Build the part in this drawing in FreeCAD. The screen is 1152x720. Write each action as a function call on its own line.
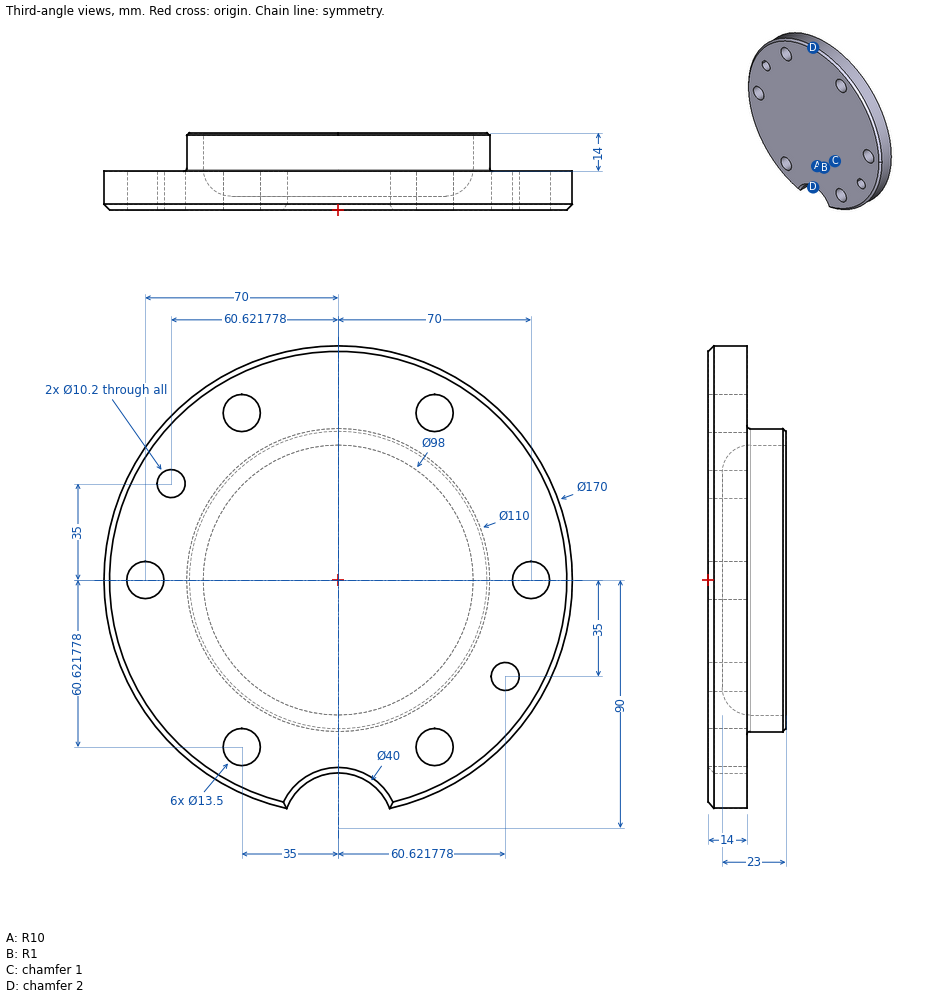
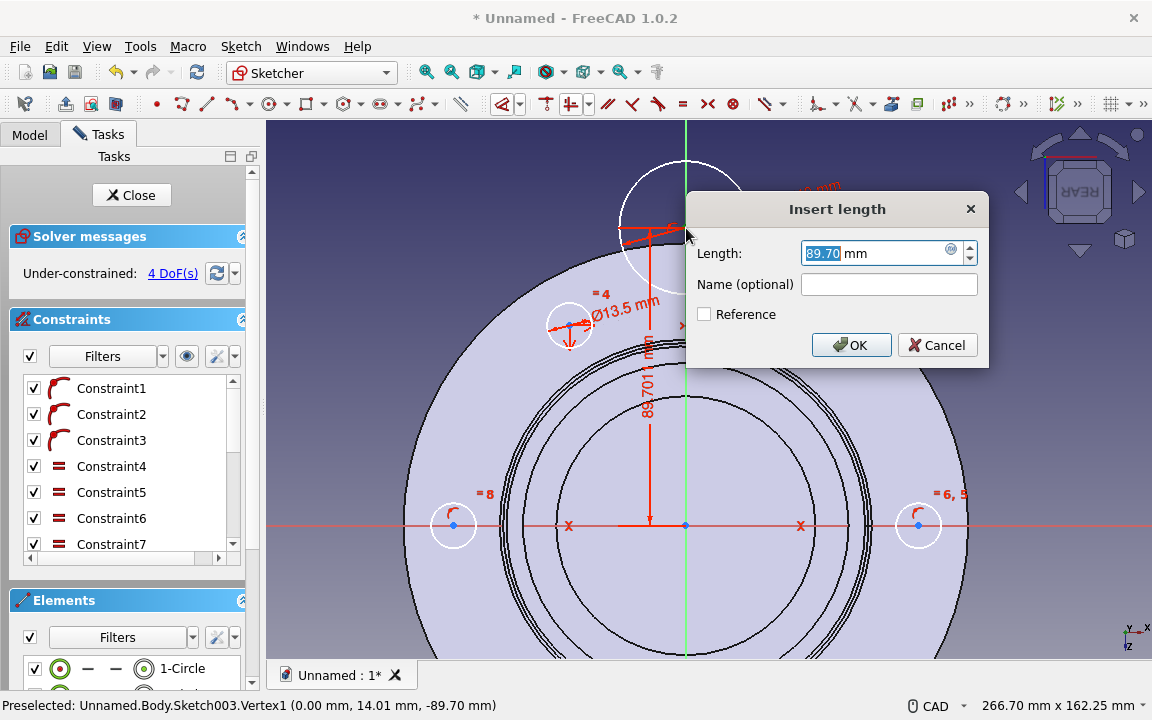
text(90)
key(Return)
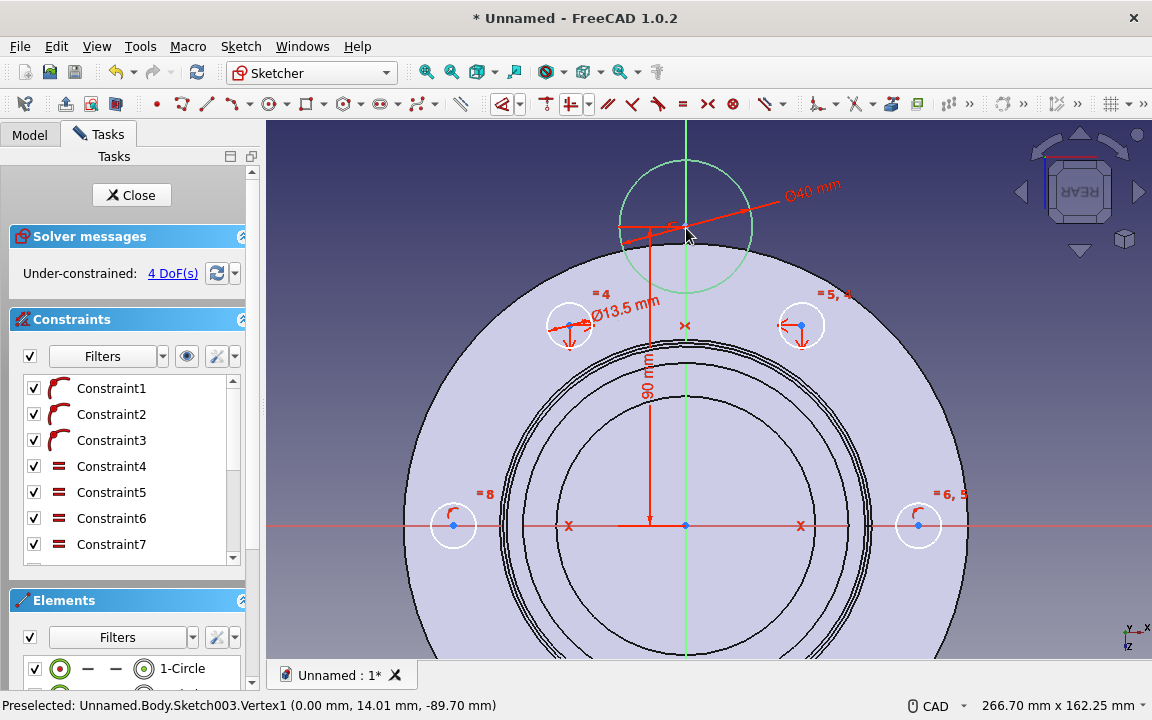
click(570, 325)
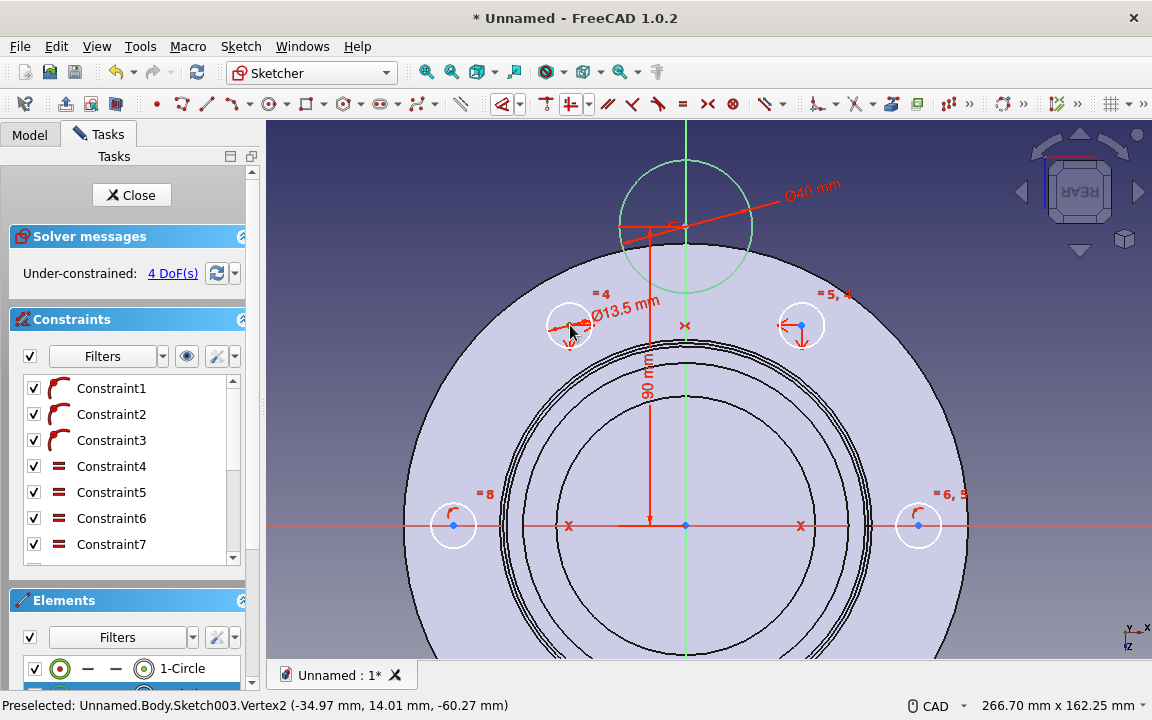
key(l)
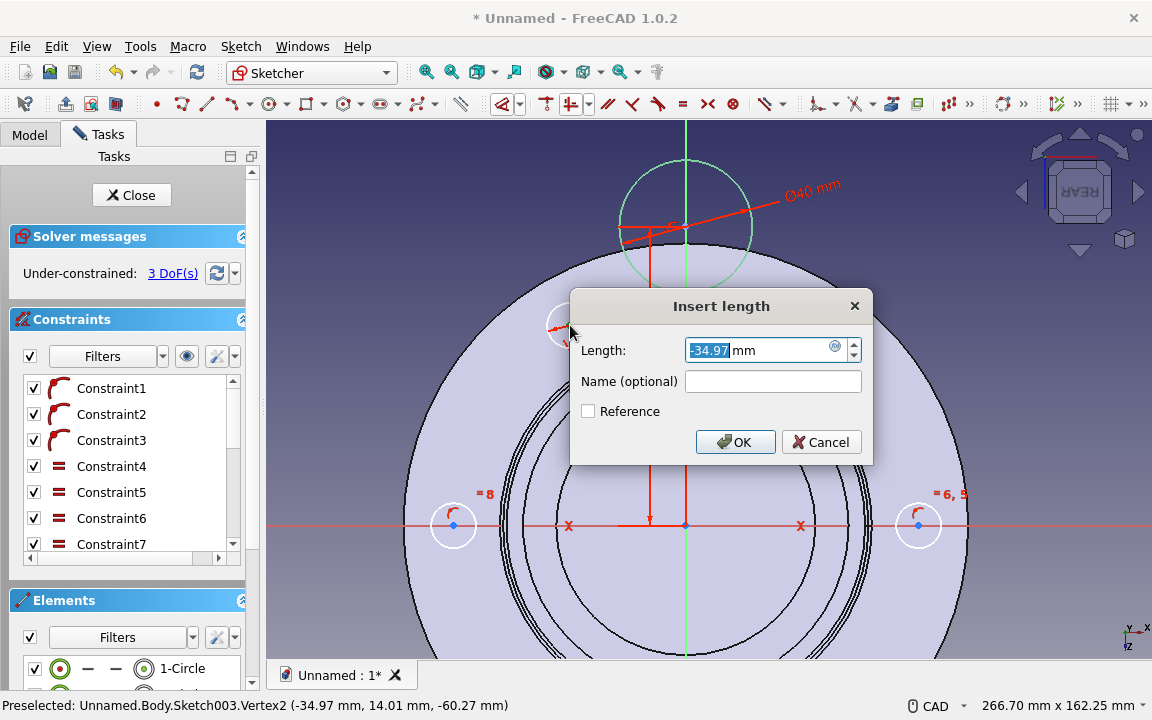
text(-35)
key(Return)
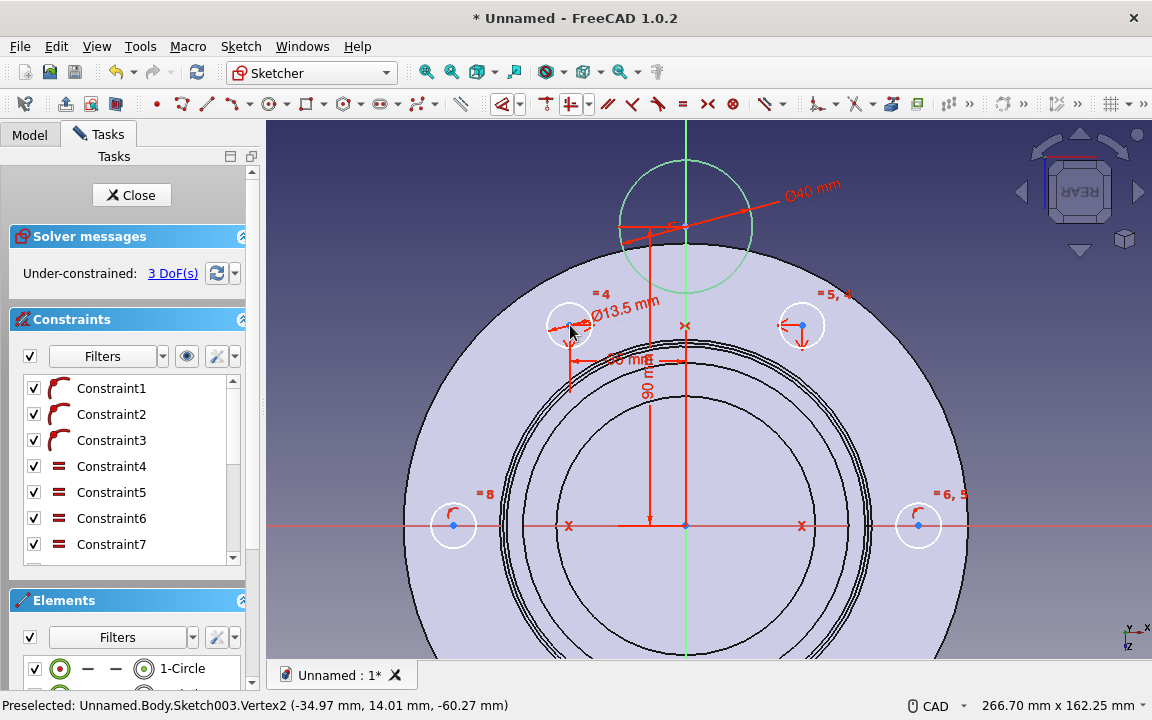
click(919, 526)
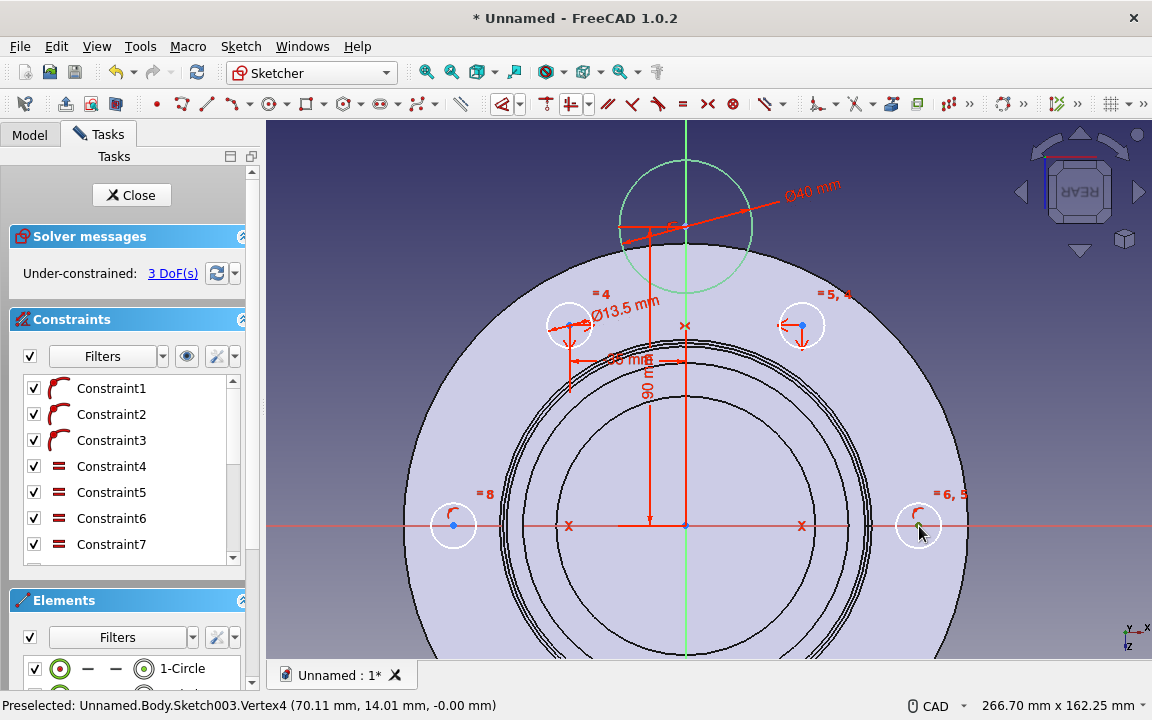
key(l)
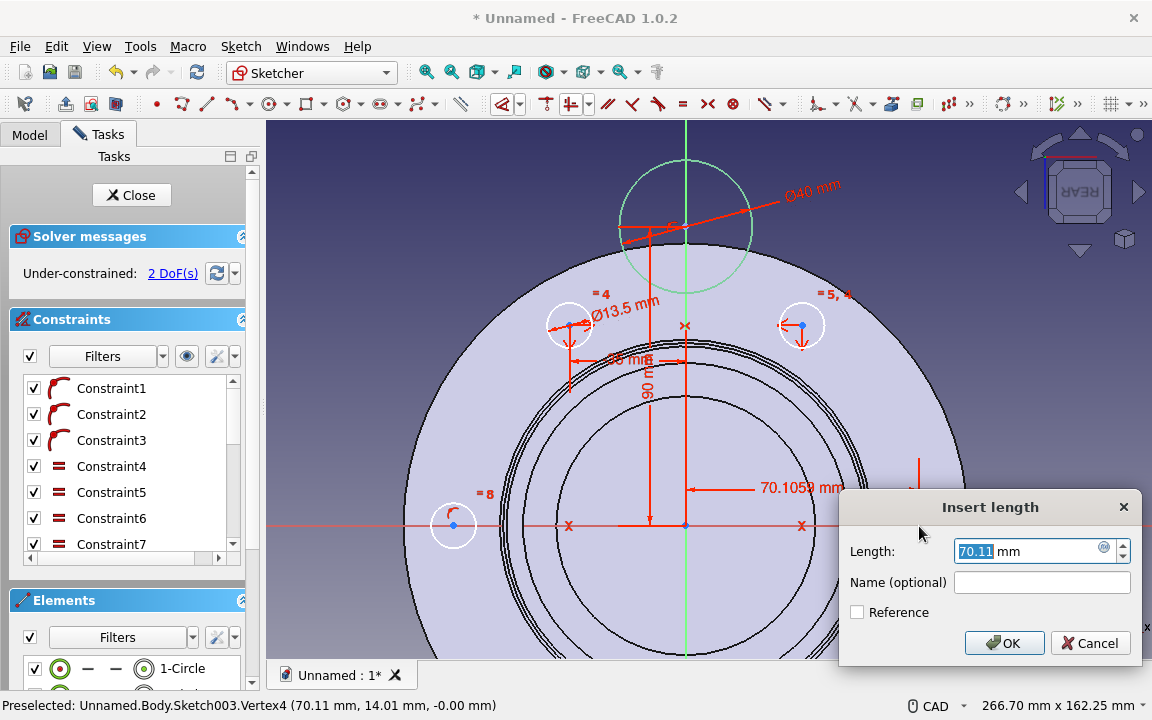
text(70)
key(Return)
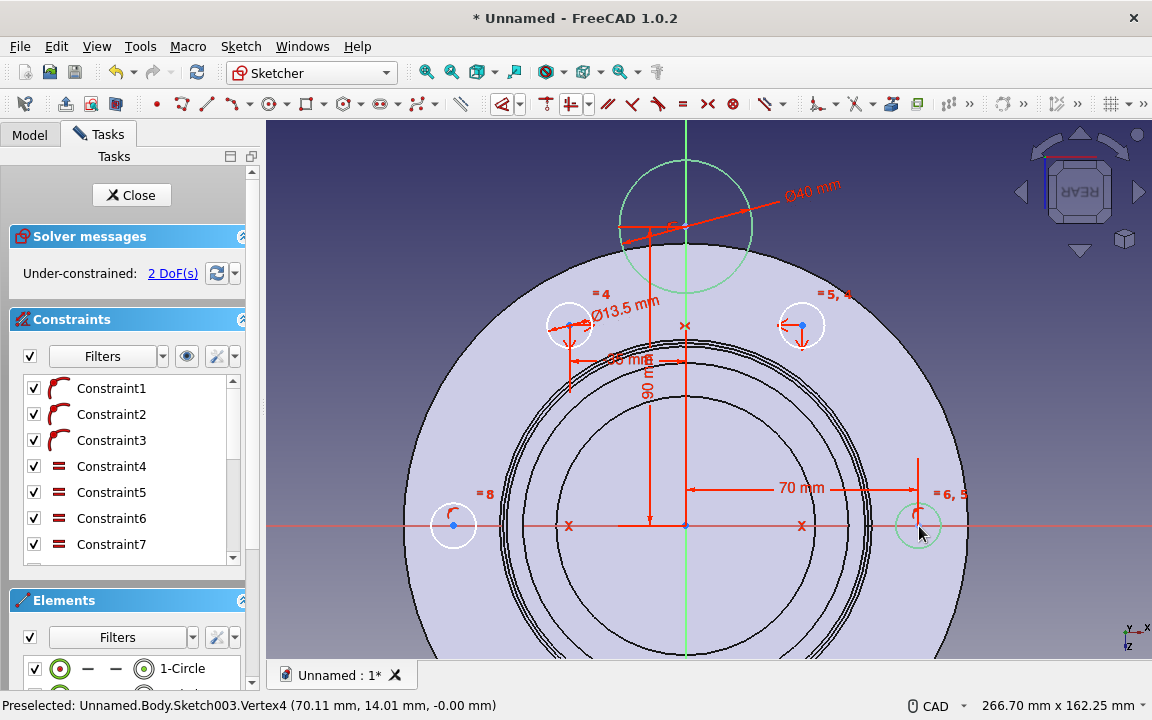
click(454, 526)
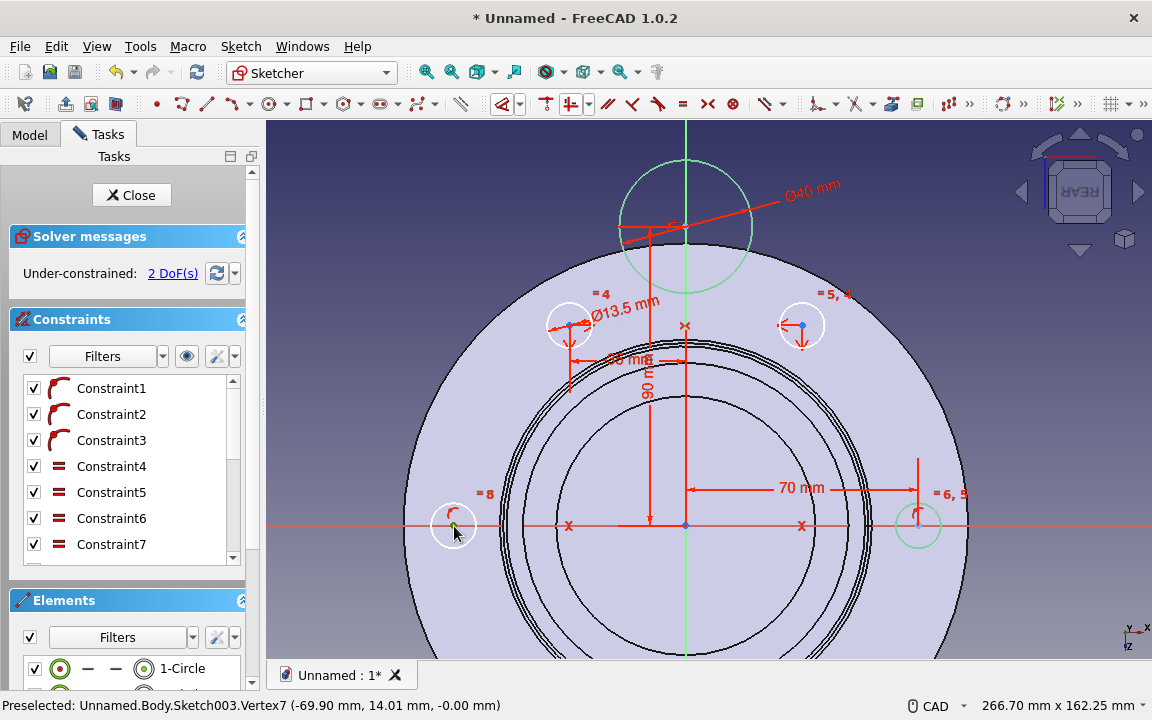
key(l)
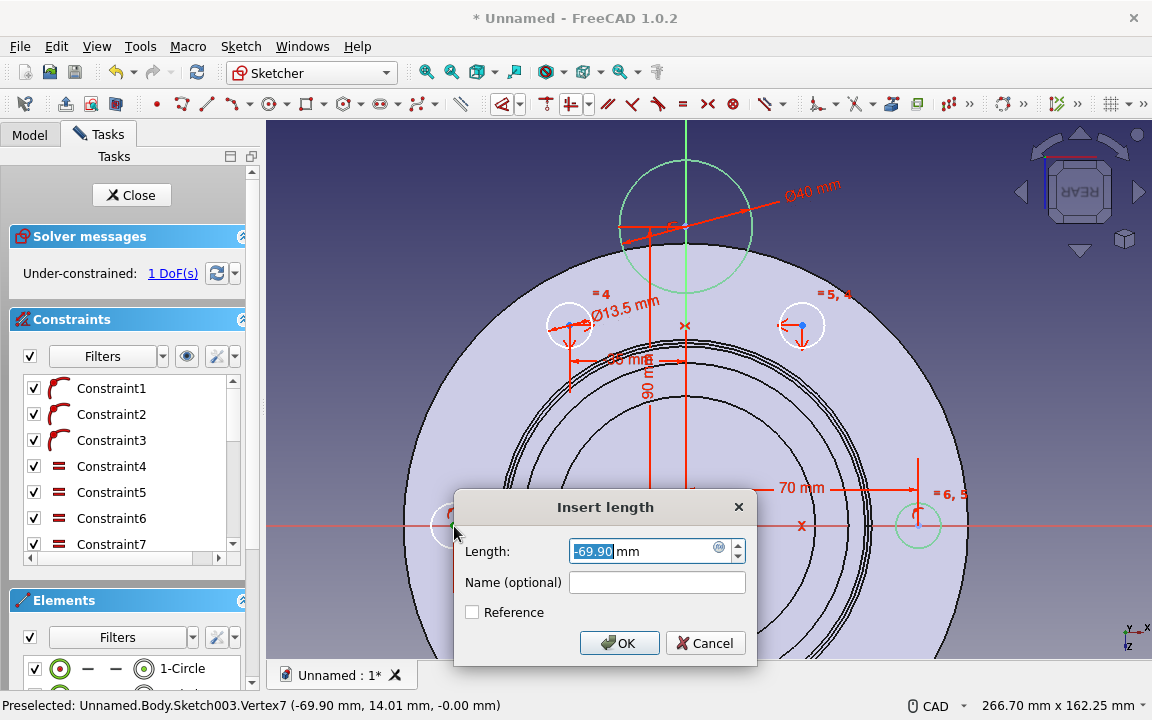
text(-70)
key(Return)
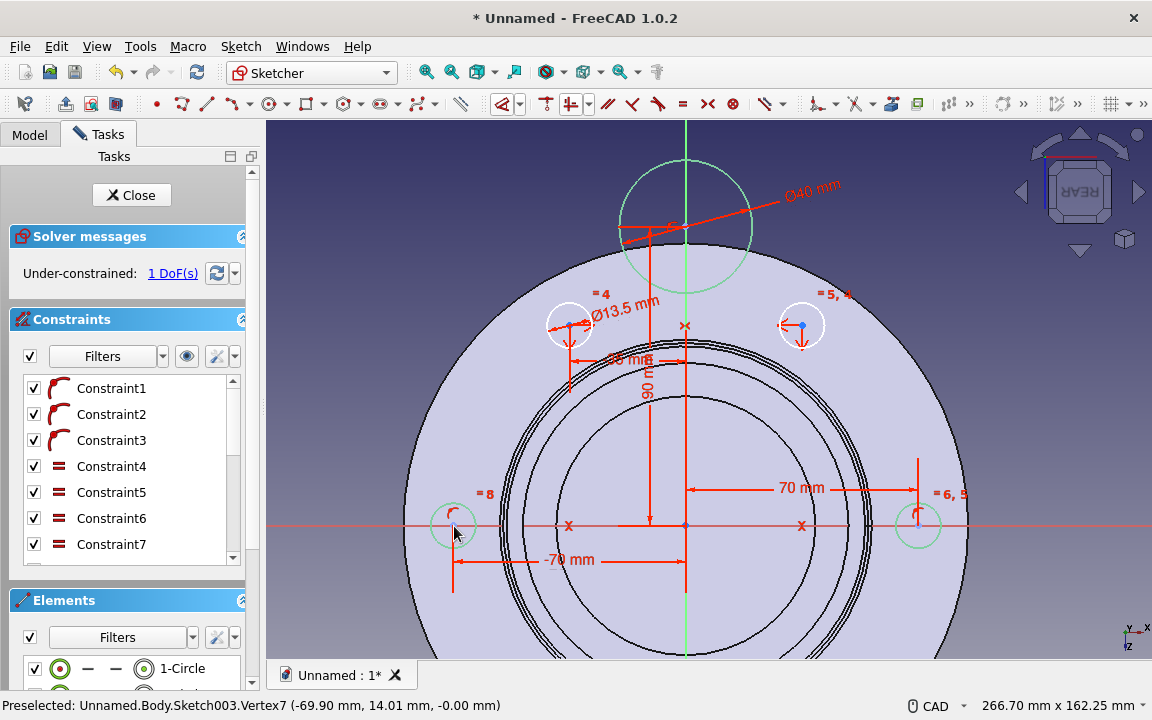
click(570, 325)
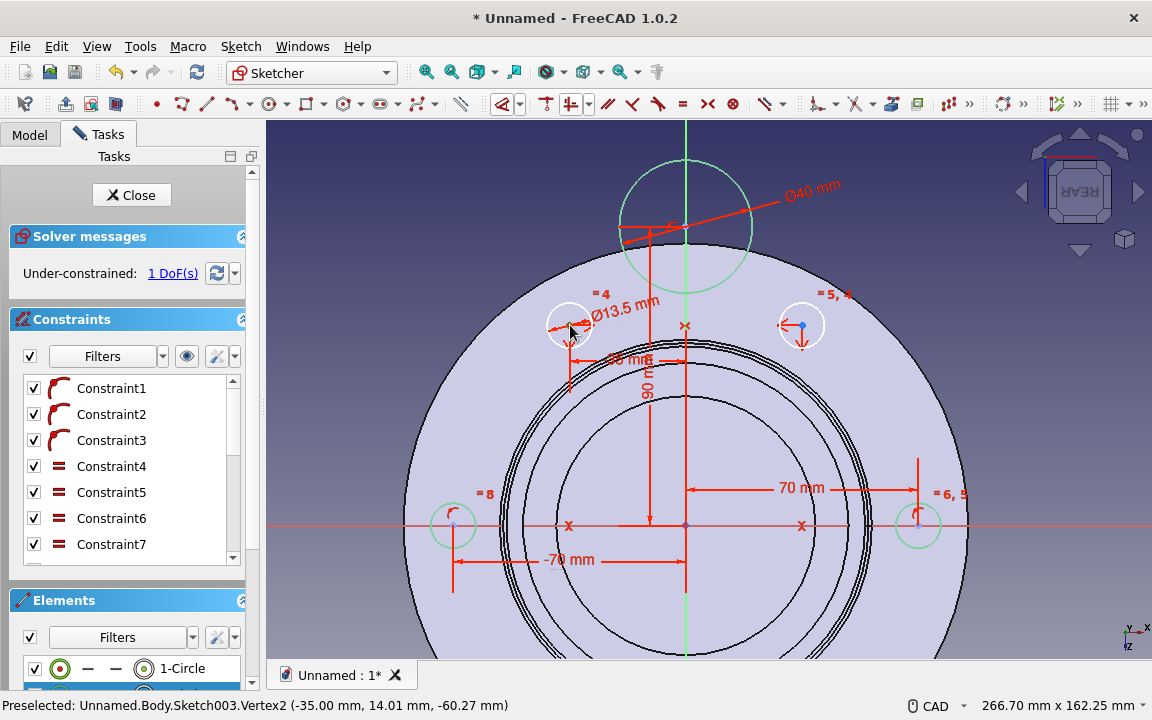
click(520, 104)